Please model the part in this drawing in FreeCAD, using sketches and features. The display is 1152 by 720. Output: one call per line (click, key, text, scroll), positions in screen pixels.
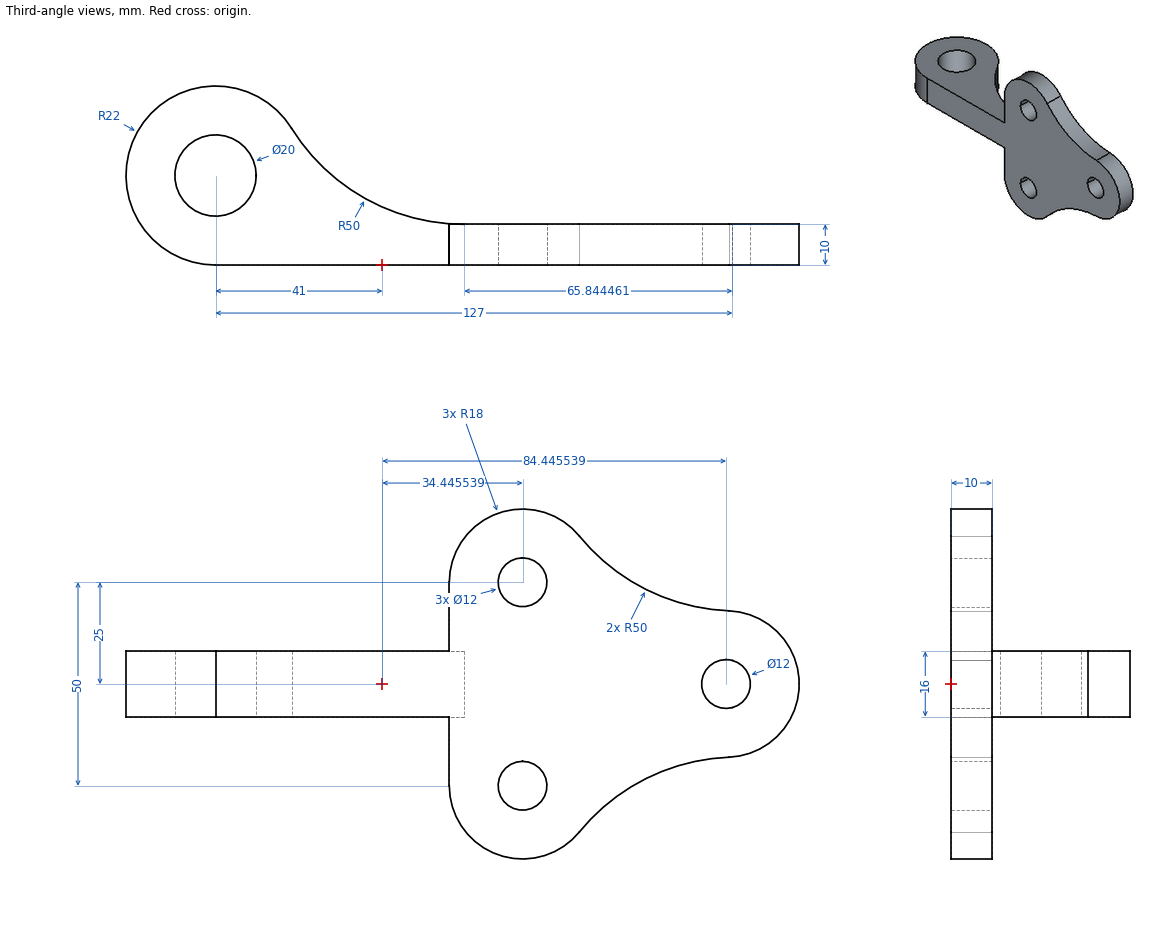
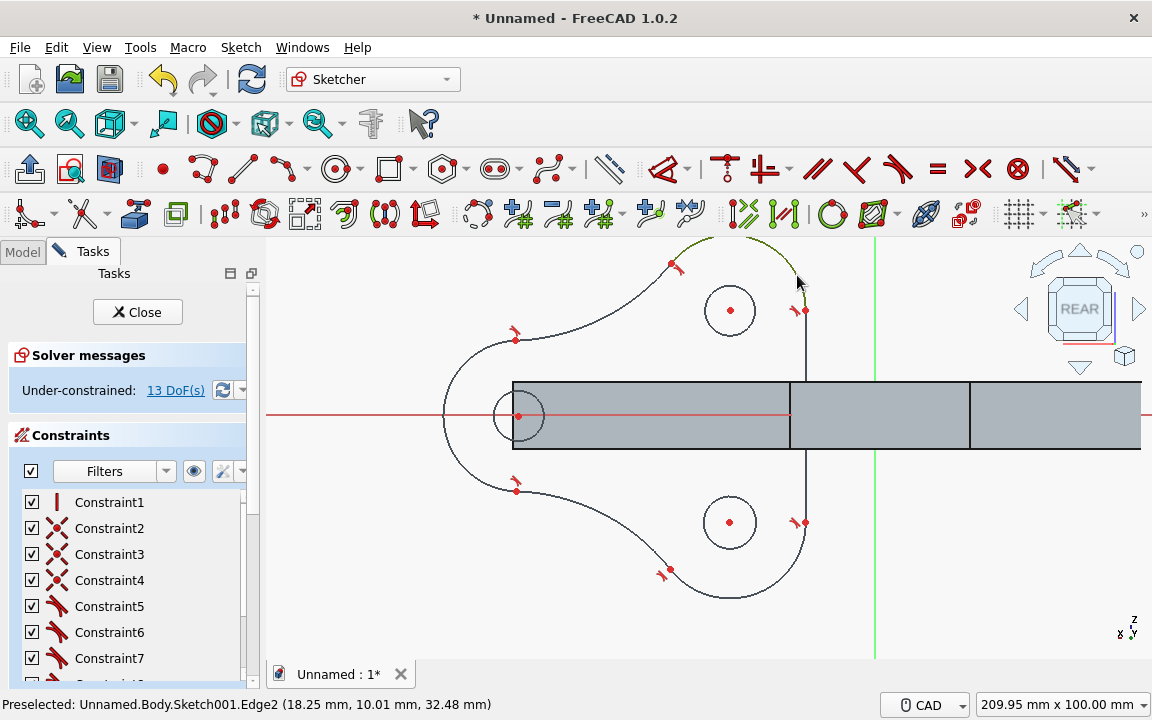
click(457, 373)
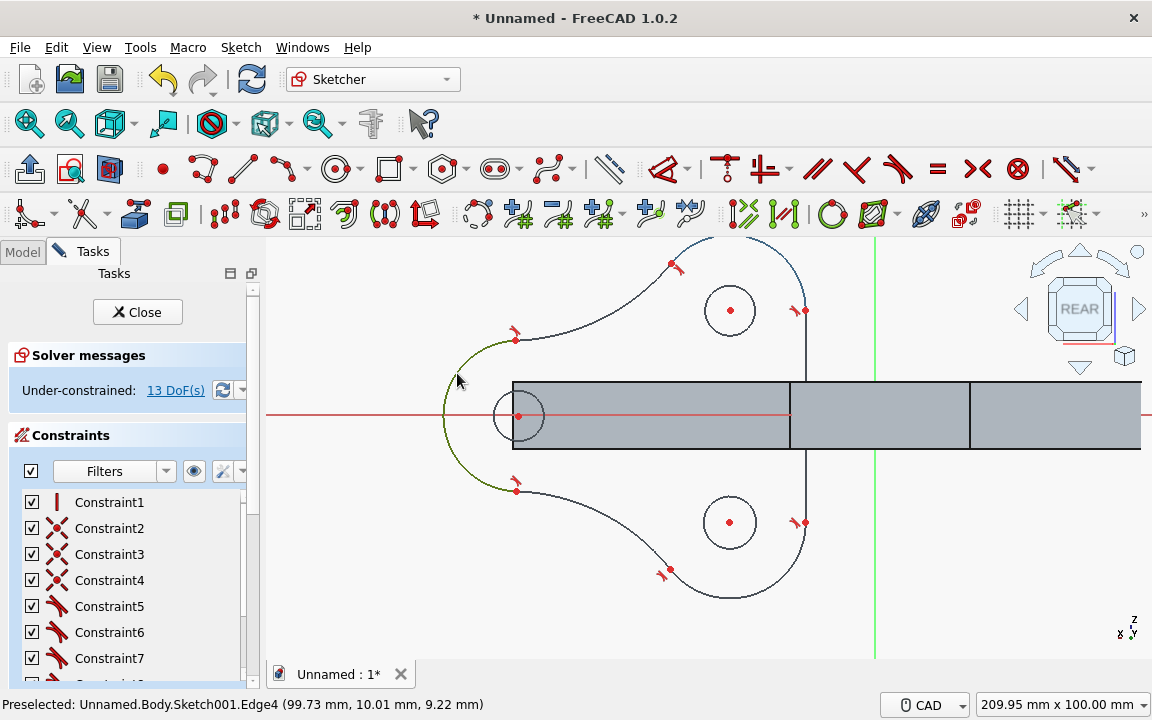
click(718, 597)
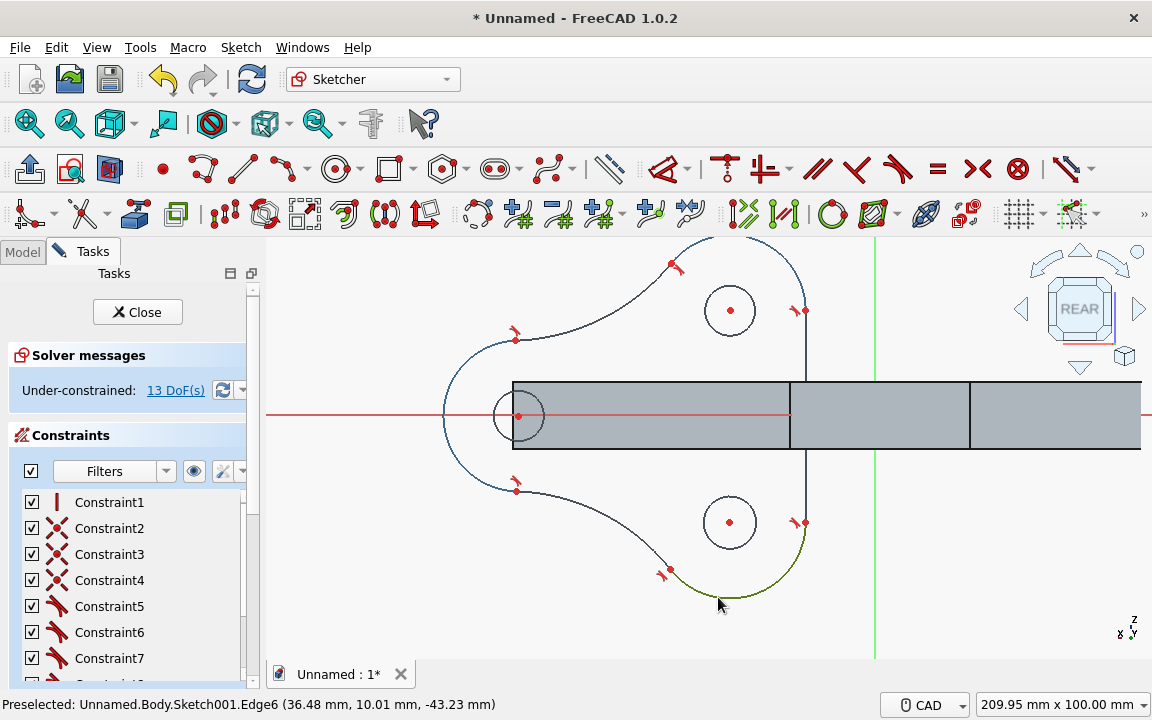
click(938, 170)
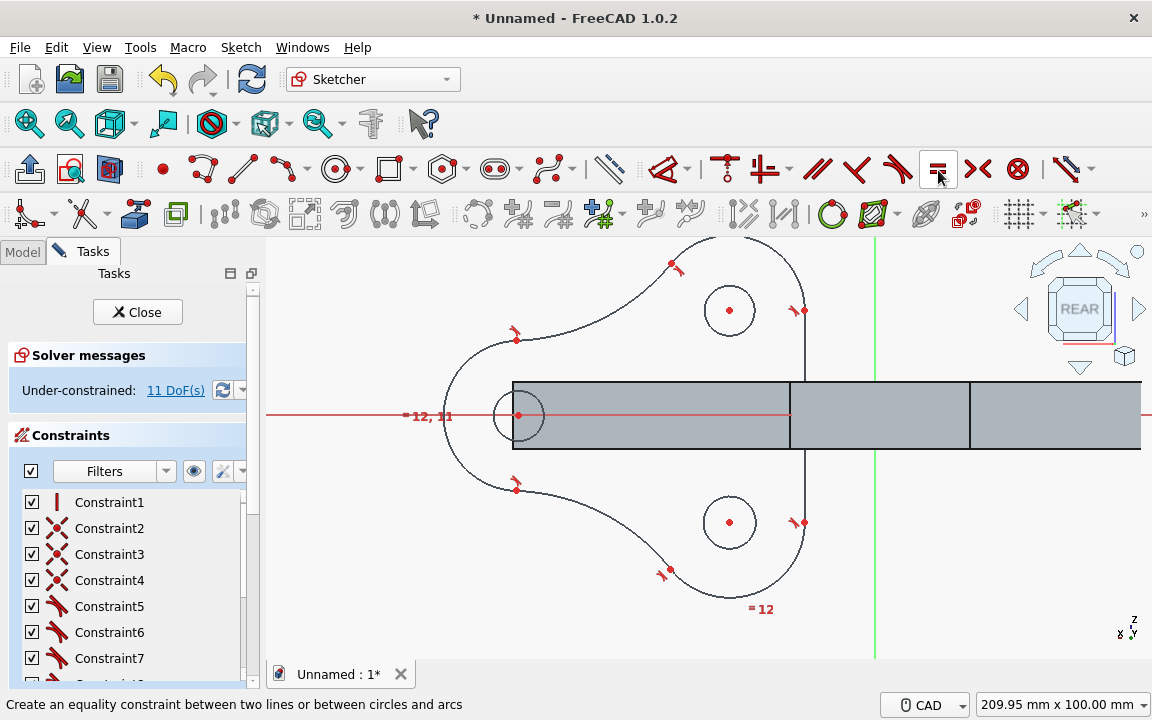
click(569, 332)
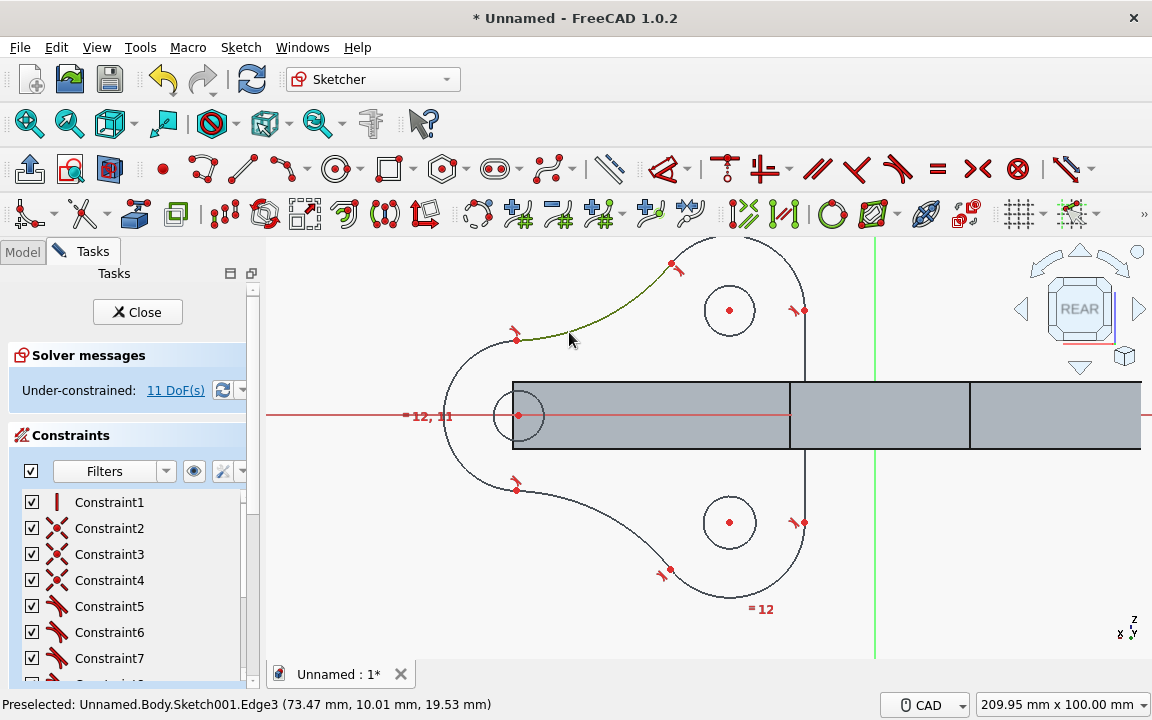
click(632, 532)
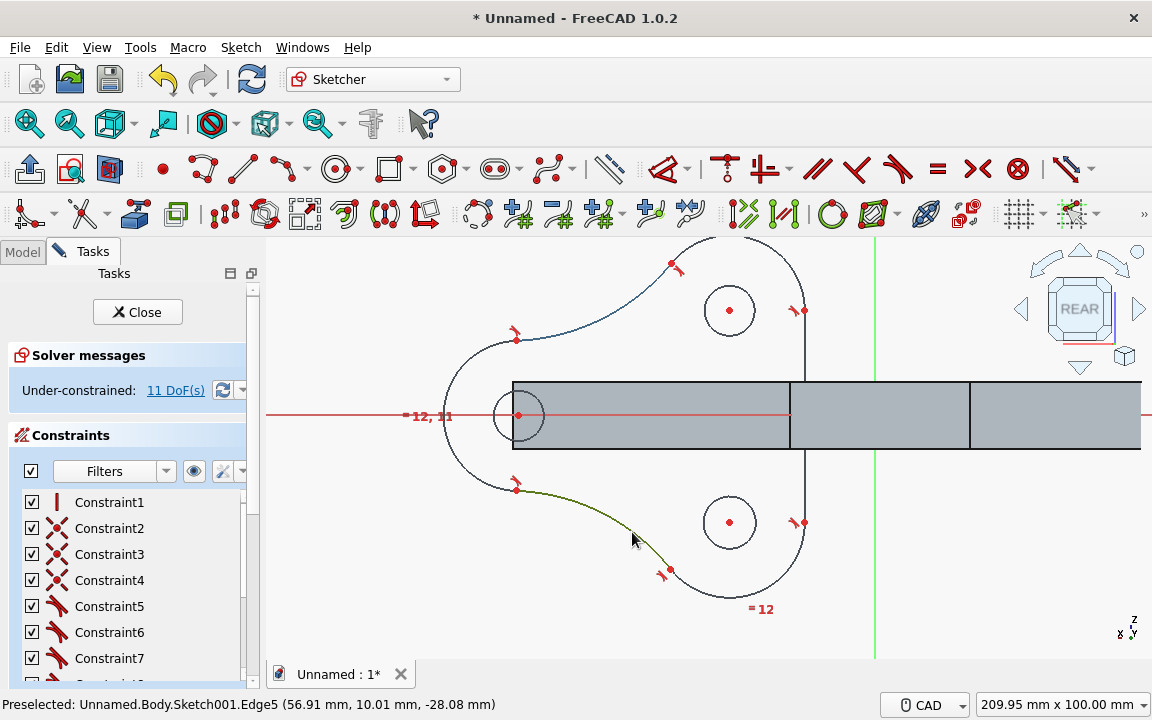
key(e)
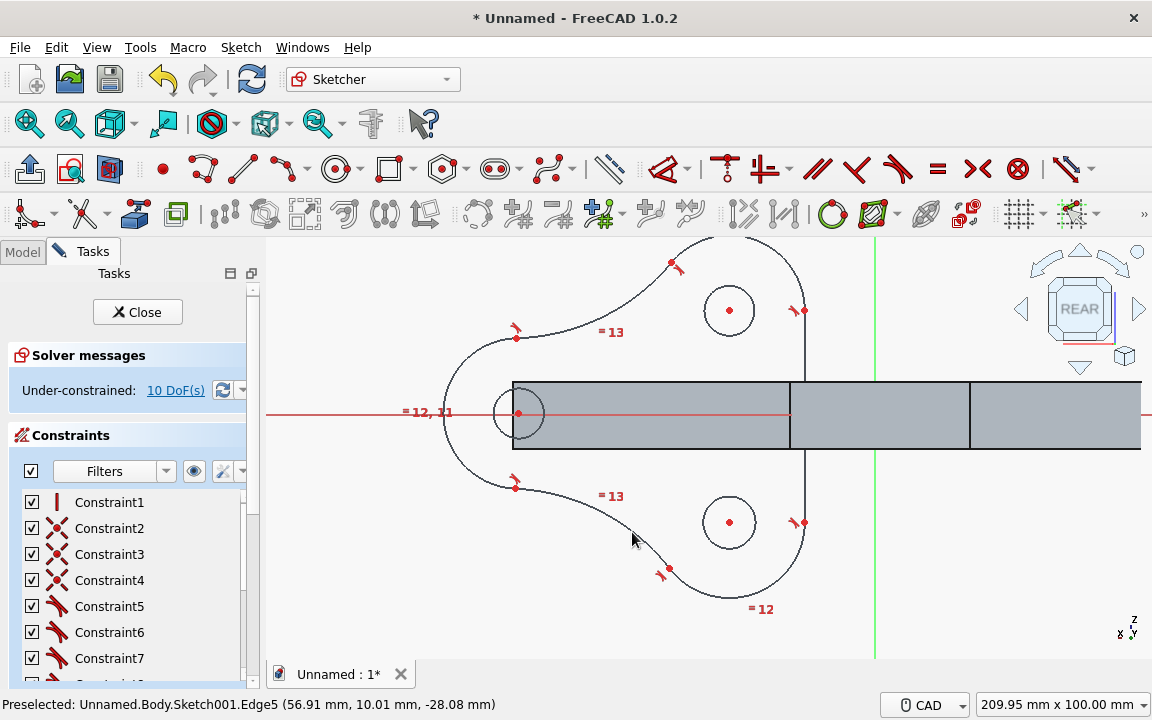
click(747, 293)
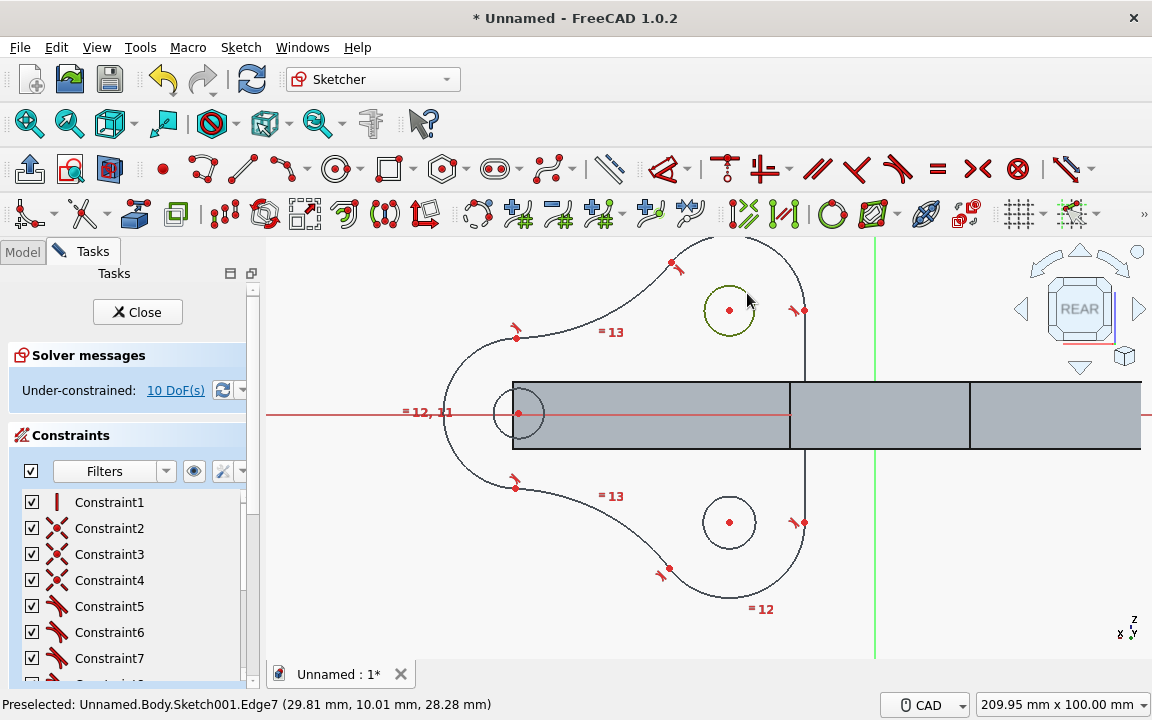
click(748, 504)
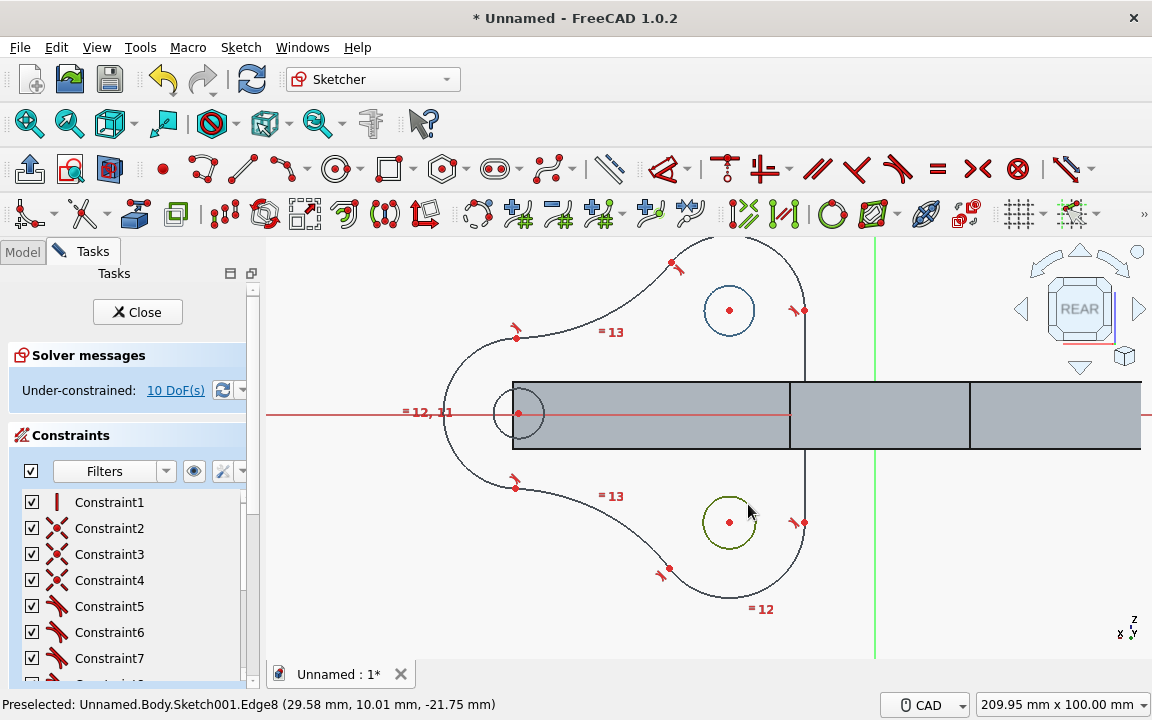
click(537, 396)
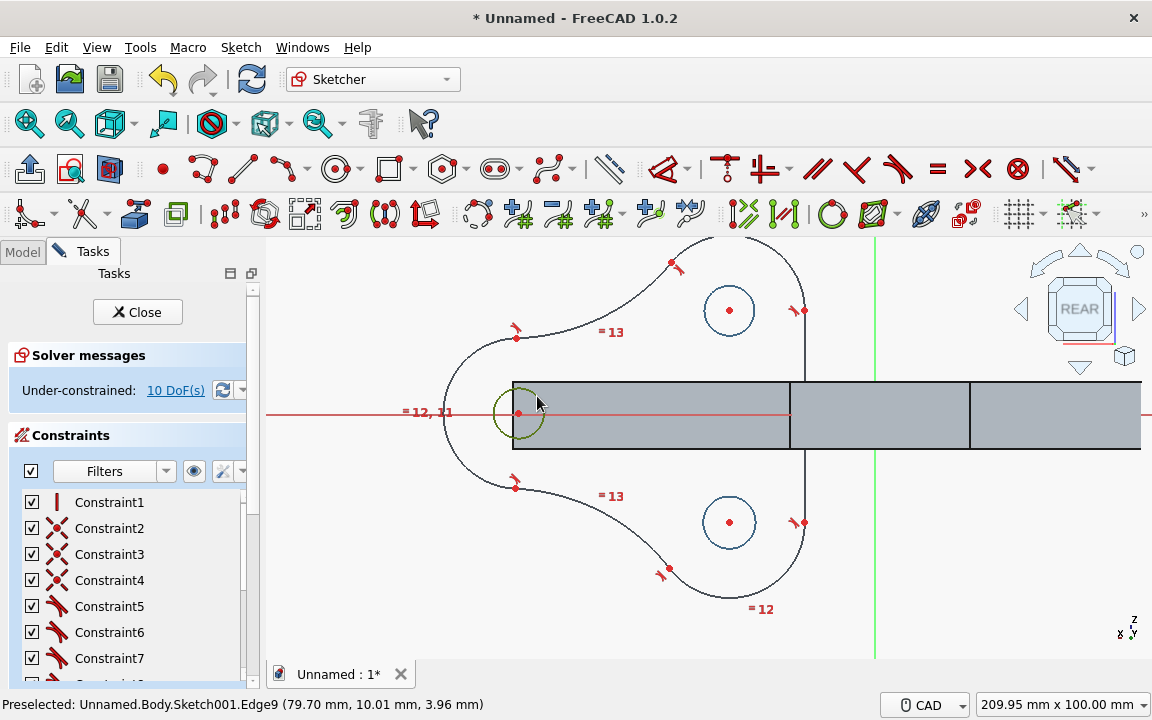
key(e)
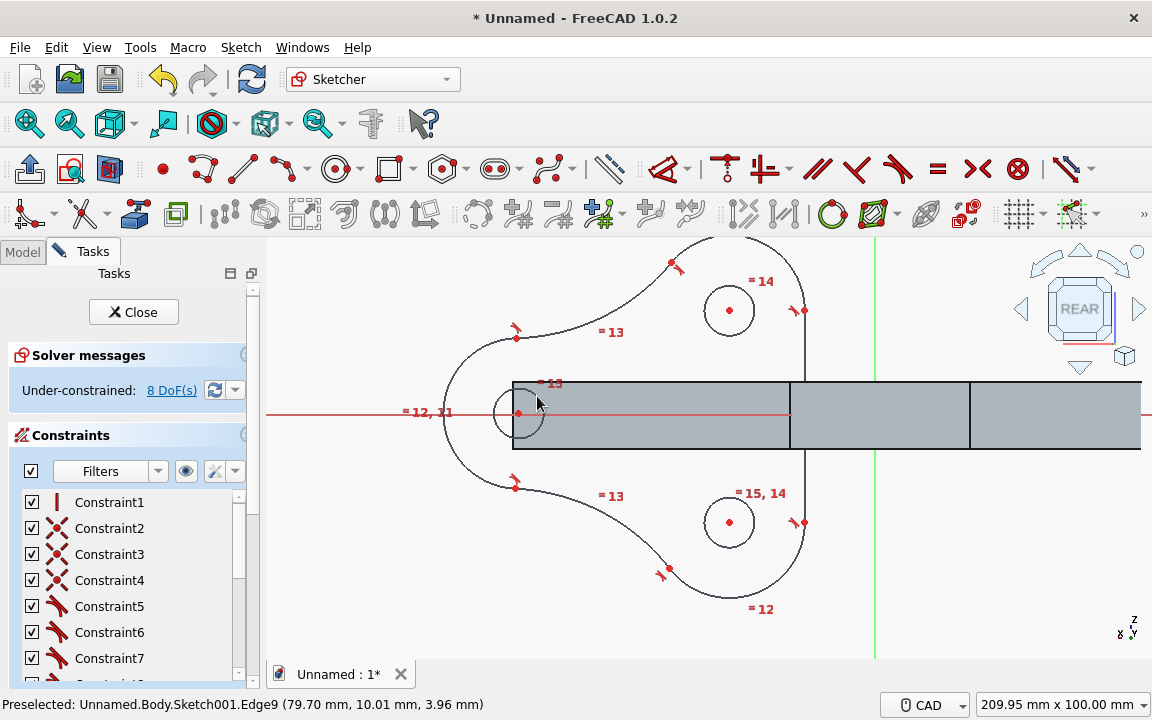
click(519, 413)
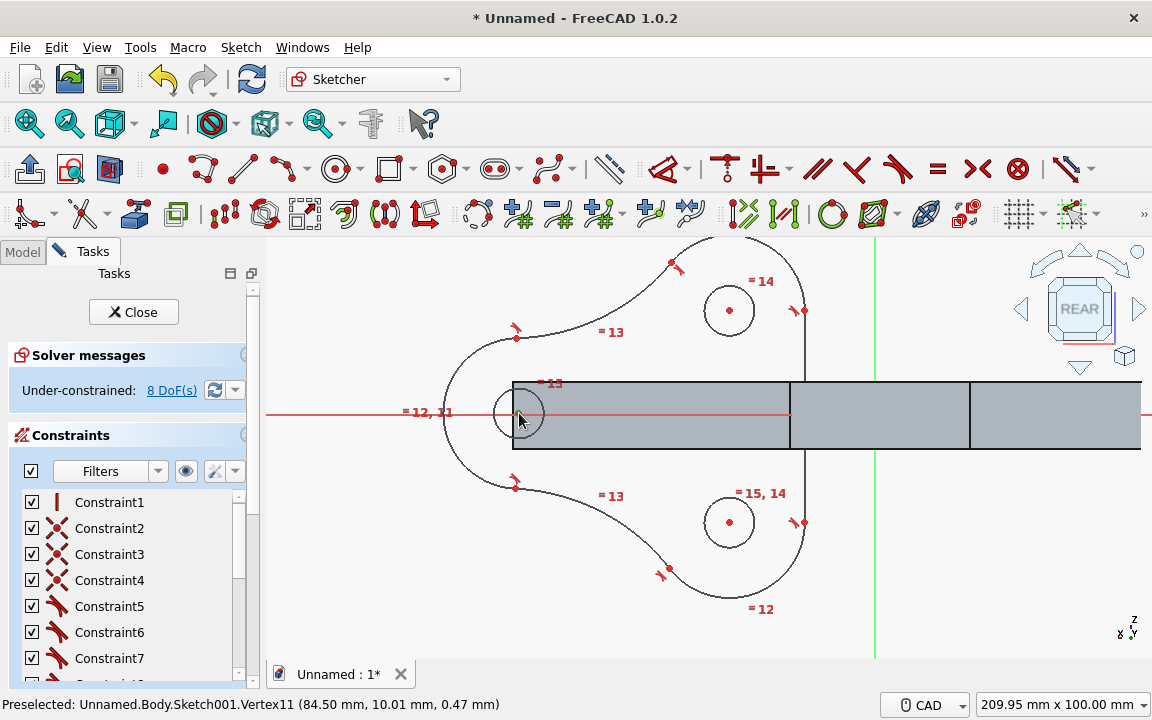
click(344, 415)